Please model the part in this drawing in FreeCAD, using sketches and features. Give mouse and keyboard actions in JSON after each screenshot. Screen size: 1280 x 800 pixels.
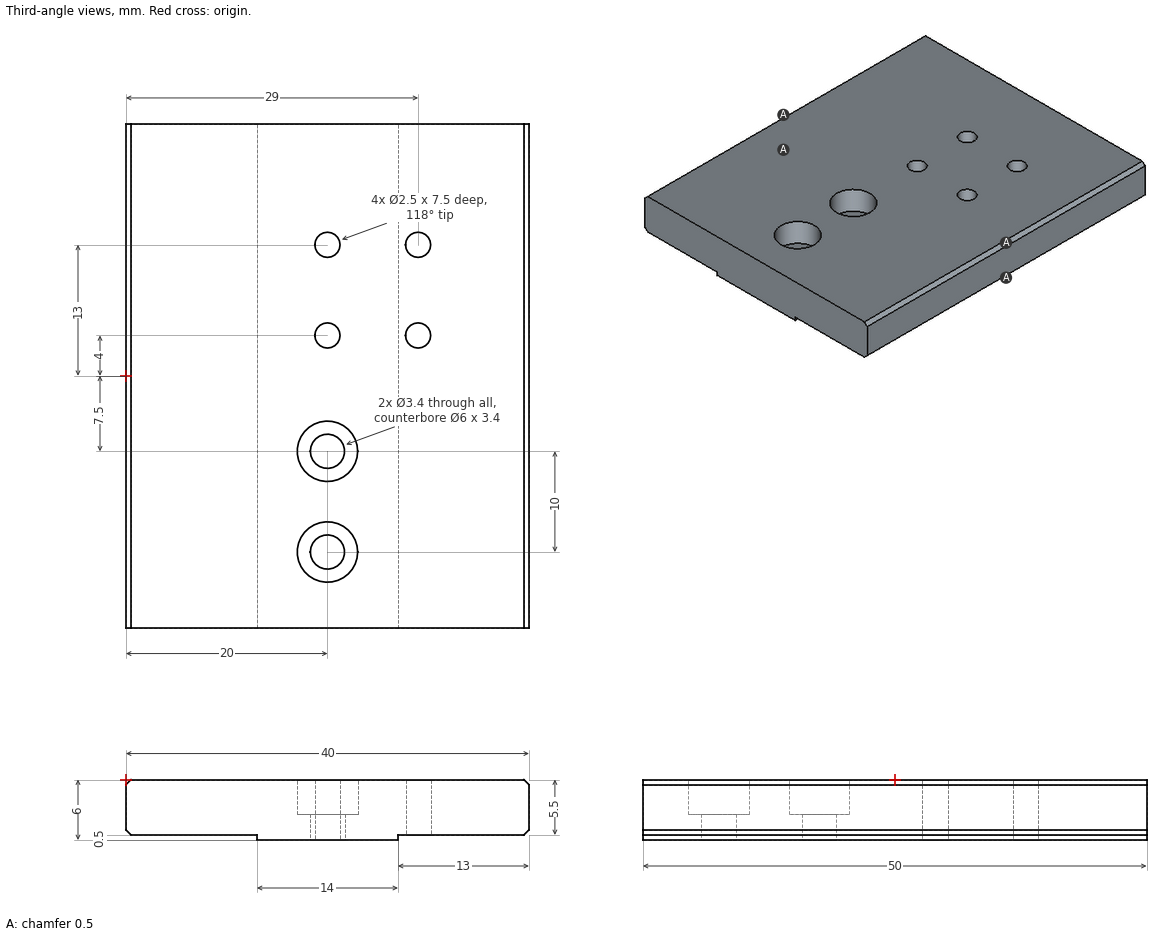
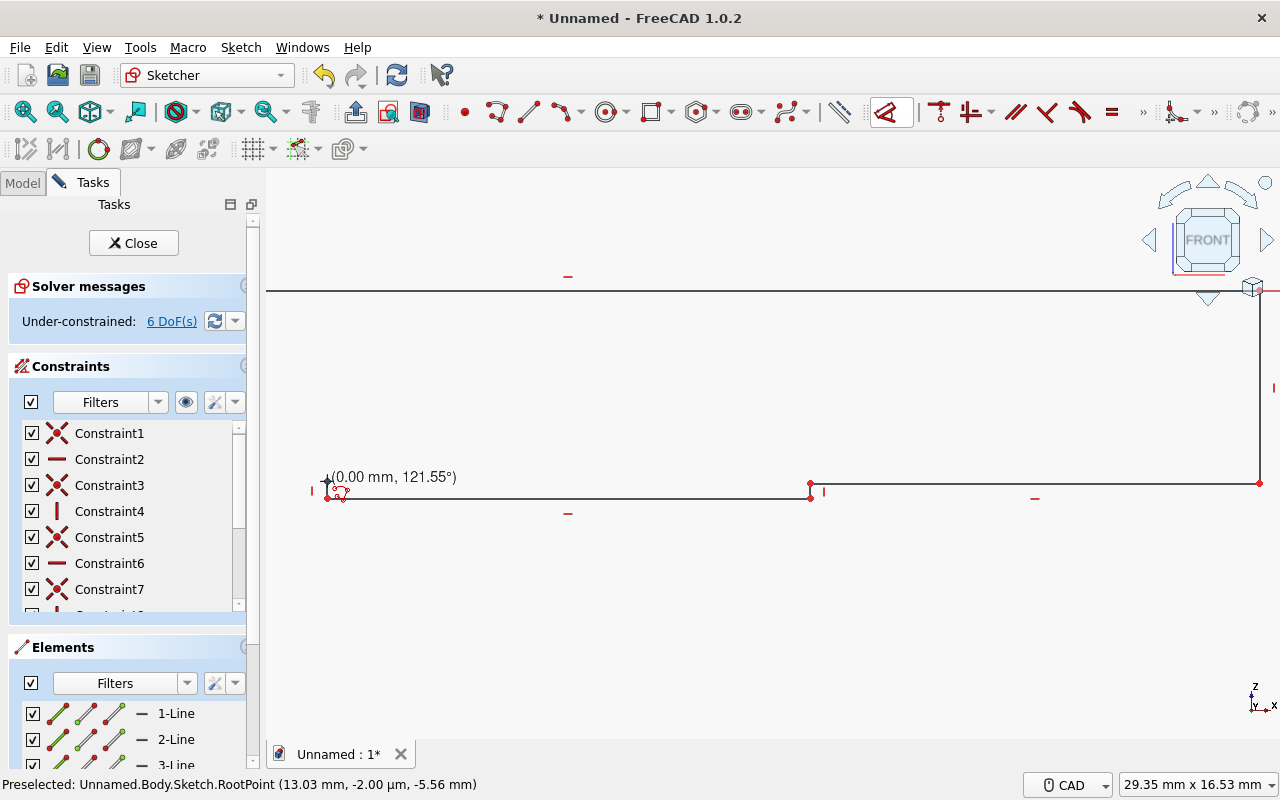
{"action": "scroll", "coordinate": [815, 502], "scroll_direction": "down", "scroll_amount": 4}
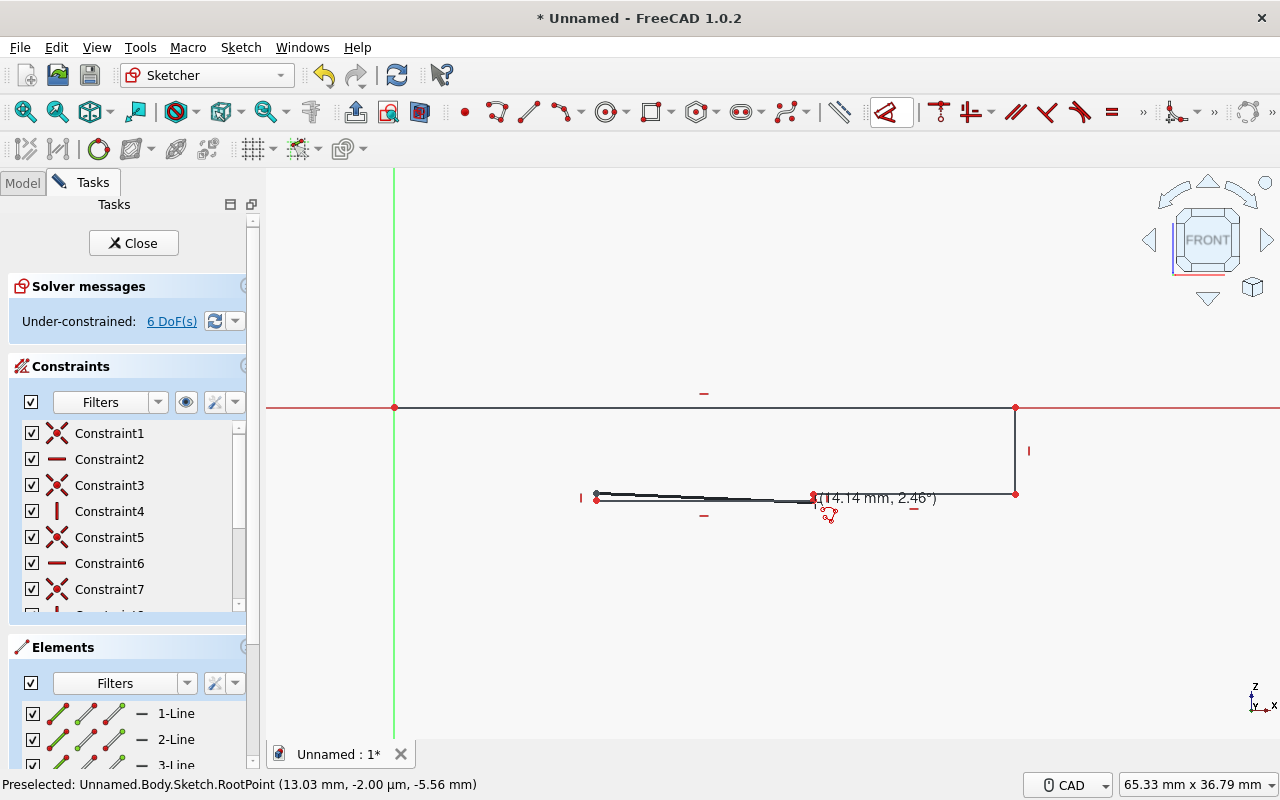
{"action": "left_click", "coordinate": [403, 493]}
{"action": "left_click", "coordinate": [394, 408]}
{"action": "key", "text": "Escape"}
{"action": "key", "text": "Escape"}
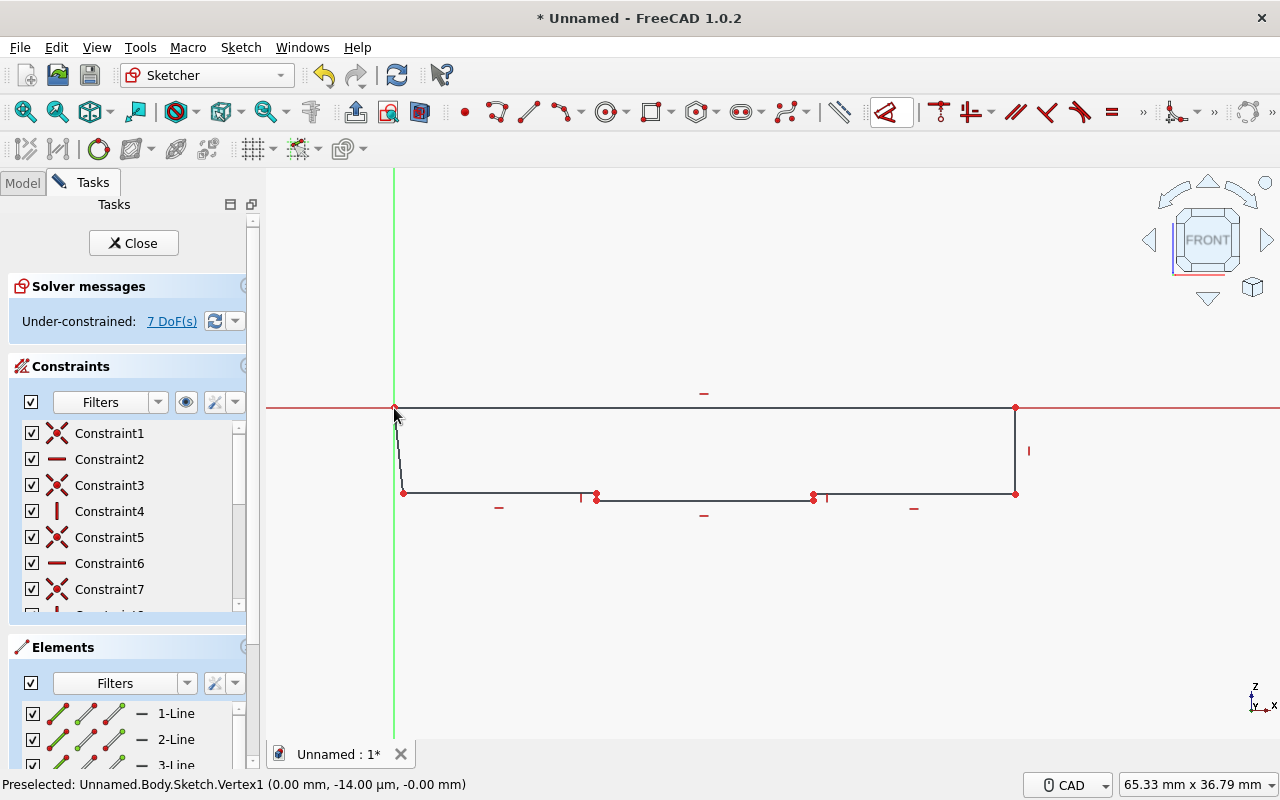
{"action": "left_click", "coordinate": [397, 433]}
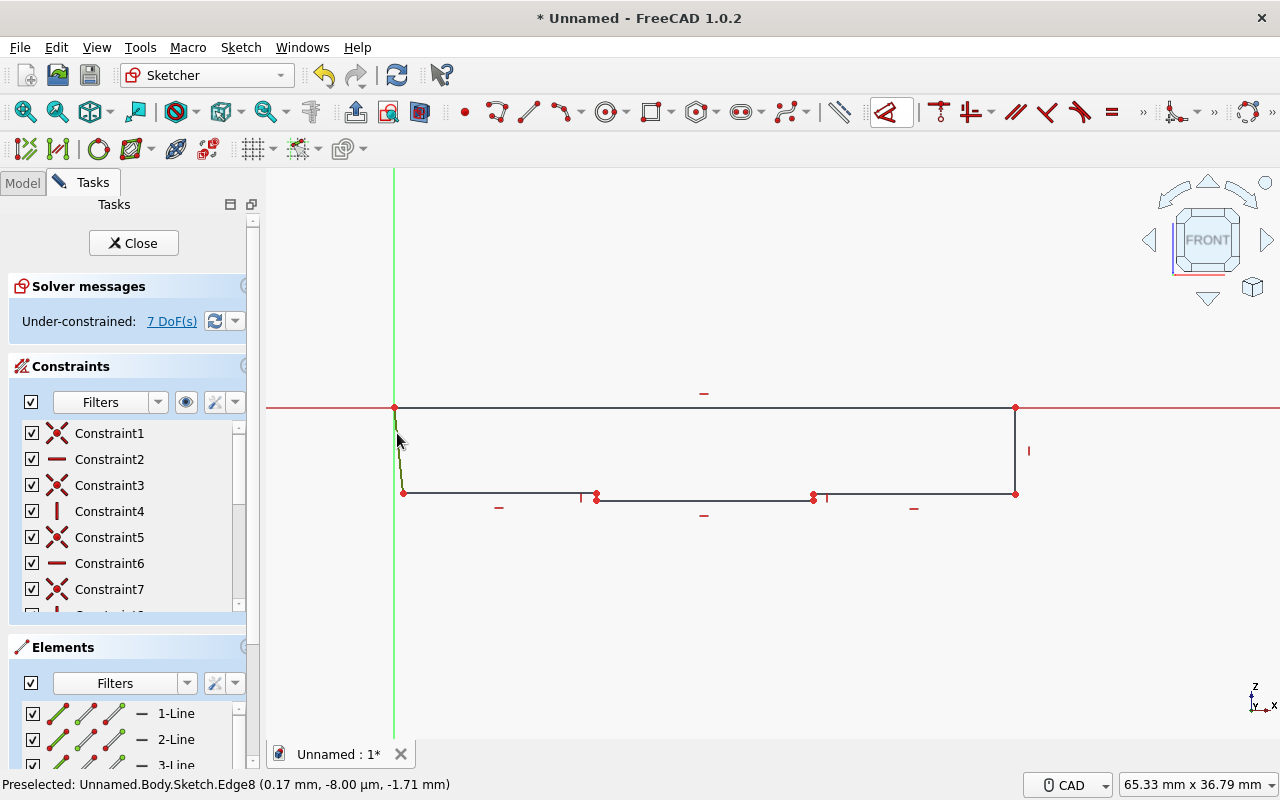
{"action": "key", "text": "v"}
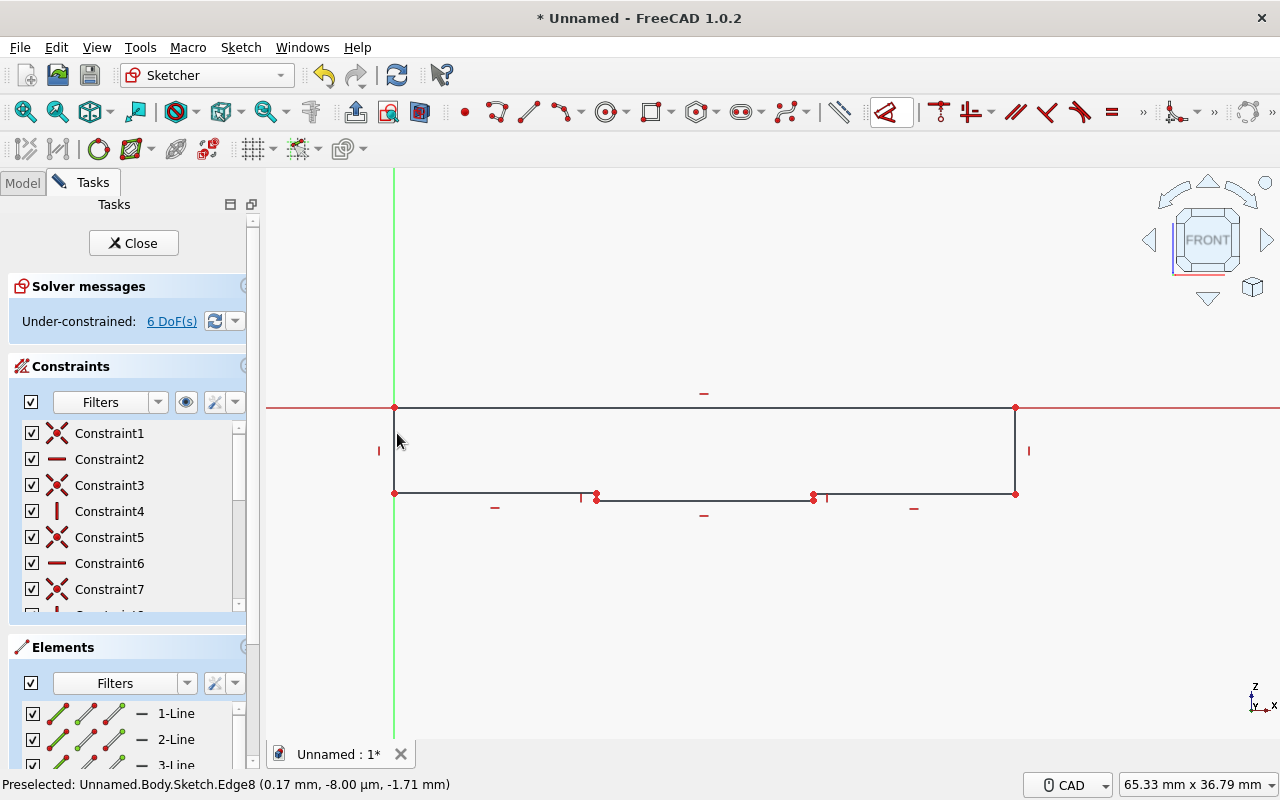
{"action": "left_click", "coordinate": [886, 112]}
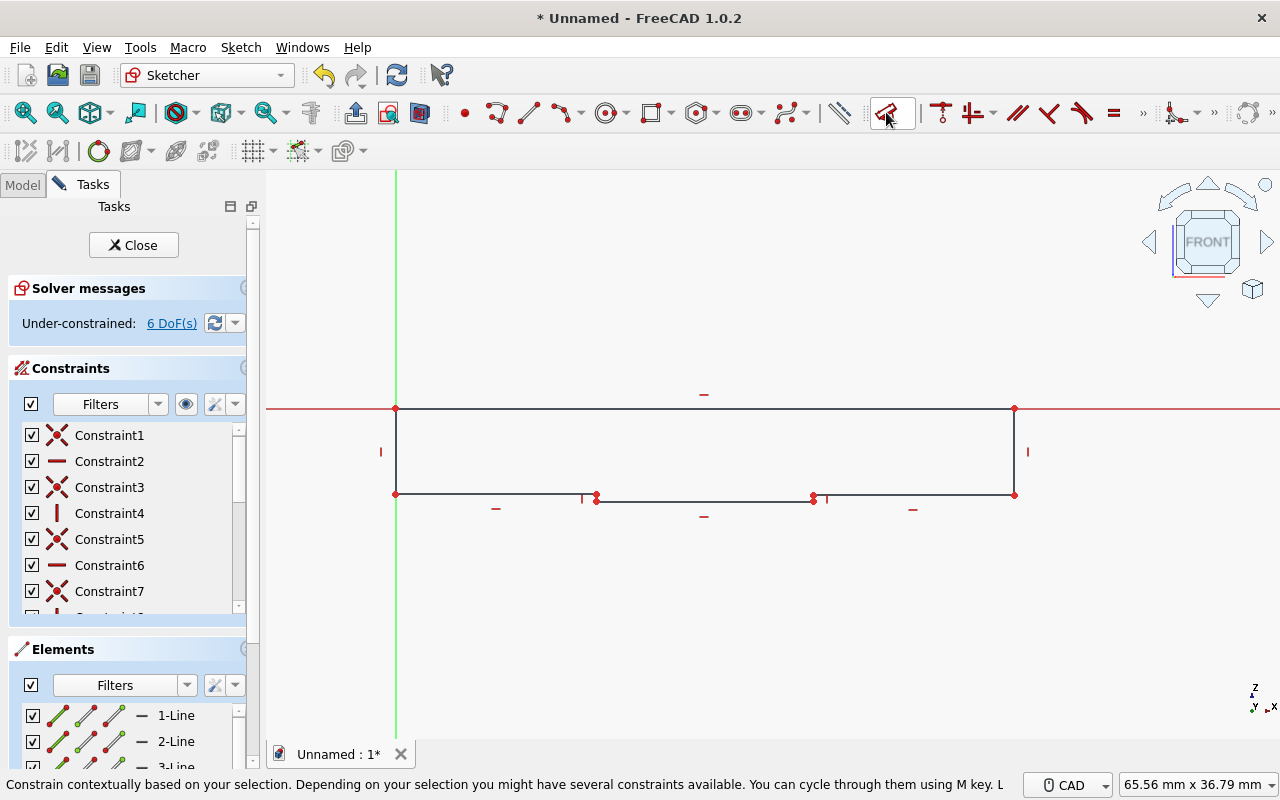
{"action": "left_click", "coordinate": [581, 409]}
{"action": "left_click", "coordinate": [705, 375]}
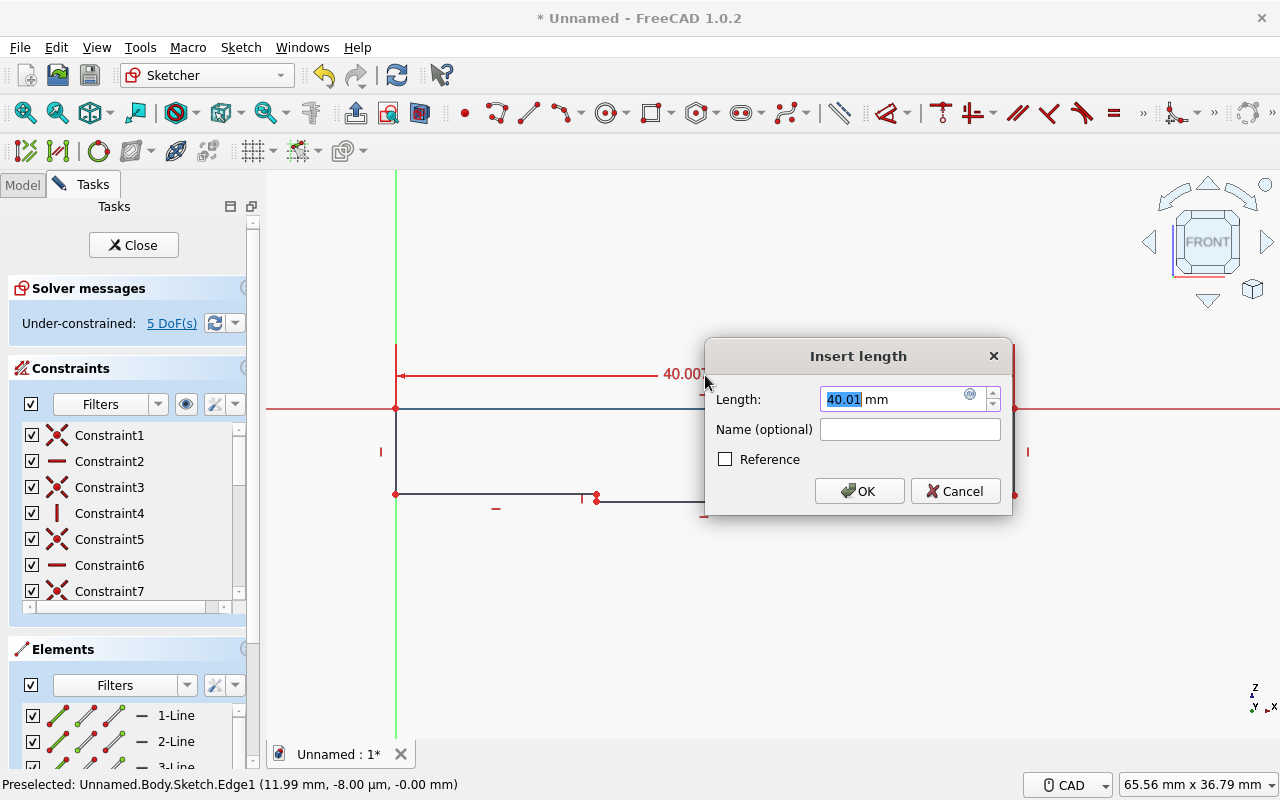
{"action": "type", "text": "40"}
{"action": "key", "text": "Return"}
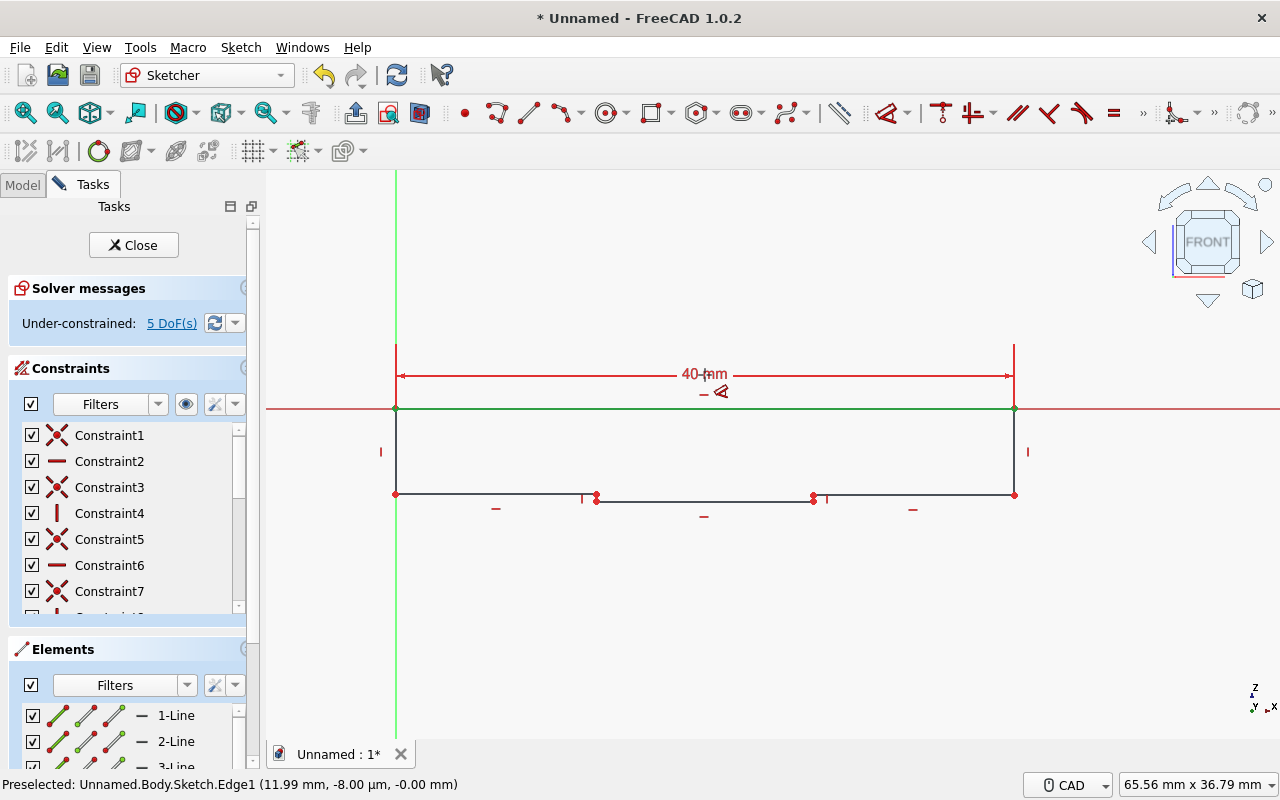
{"action": "left_click", "coordinate": [954, 495]}
{"action": "left_click", "coordinate": [914, 529]}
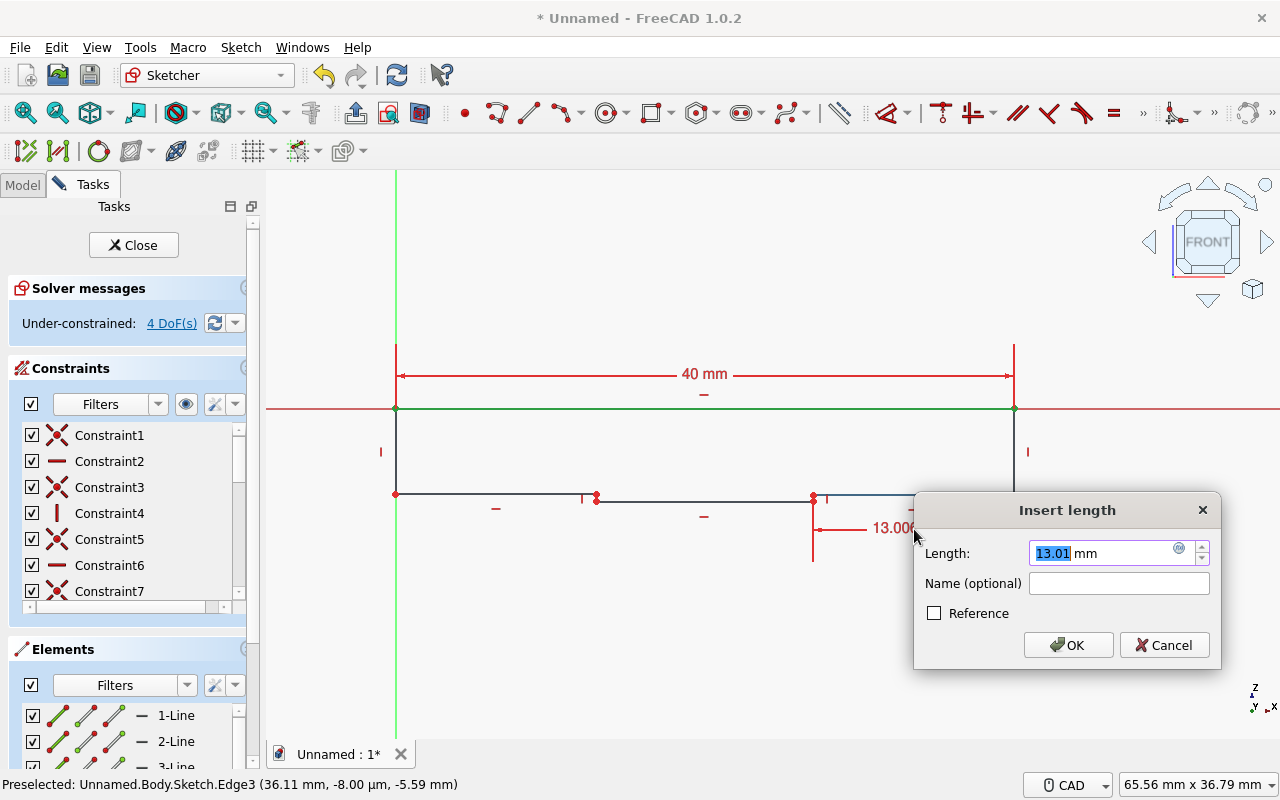
{"action": "type", "text": "13"}
{"action": "key", "text": "Return"}